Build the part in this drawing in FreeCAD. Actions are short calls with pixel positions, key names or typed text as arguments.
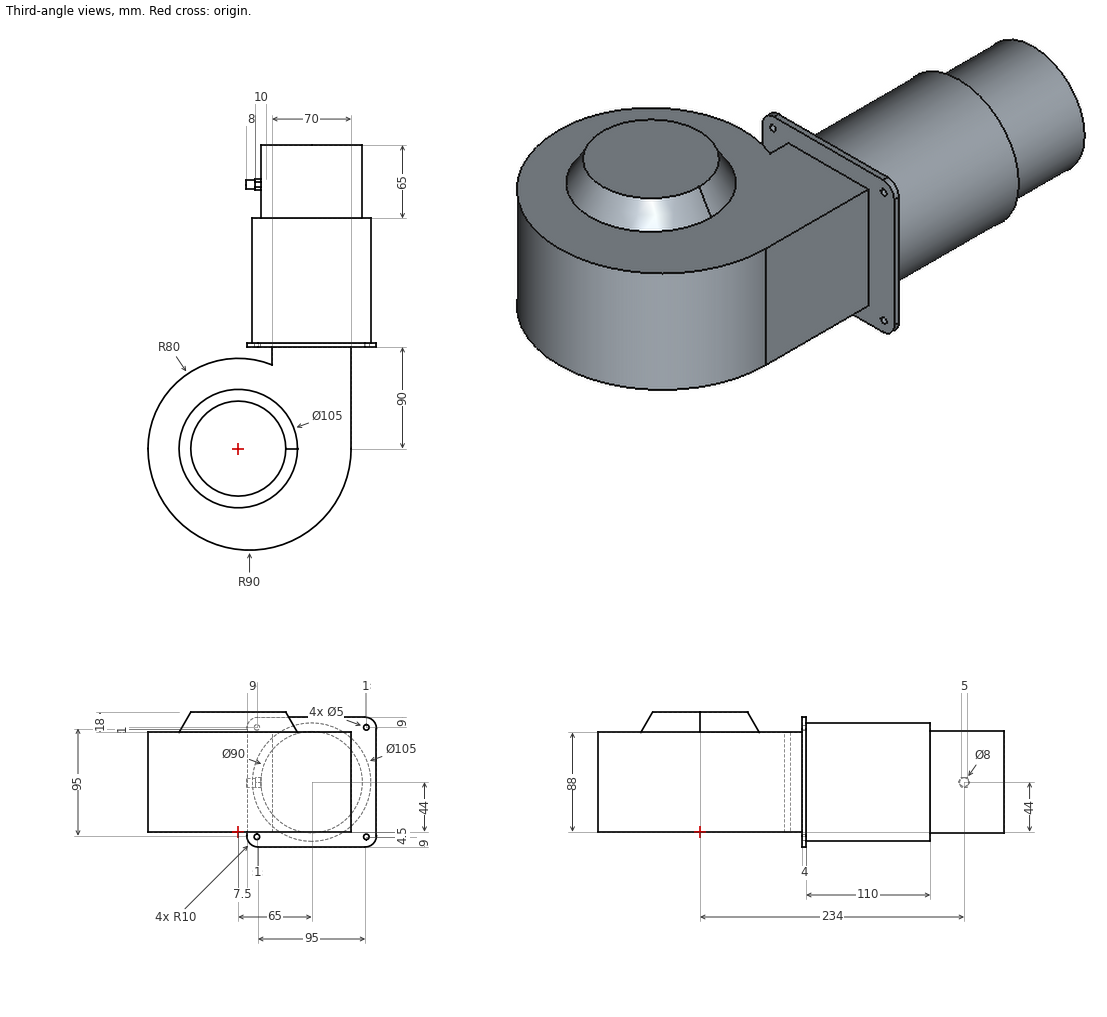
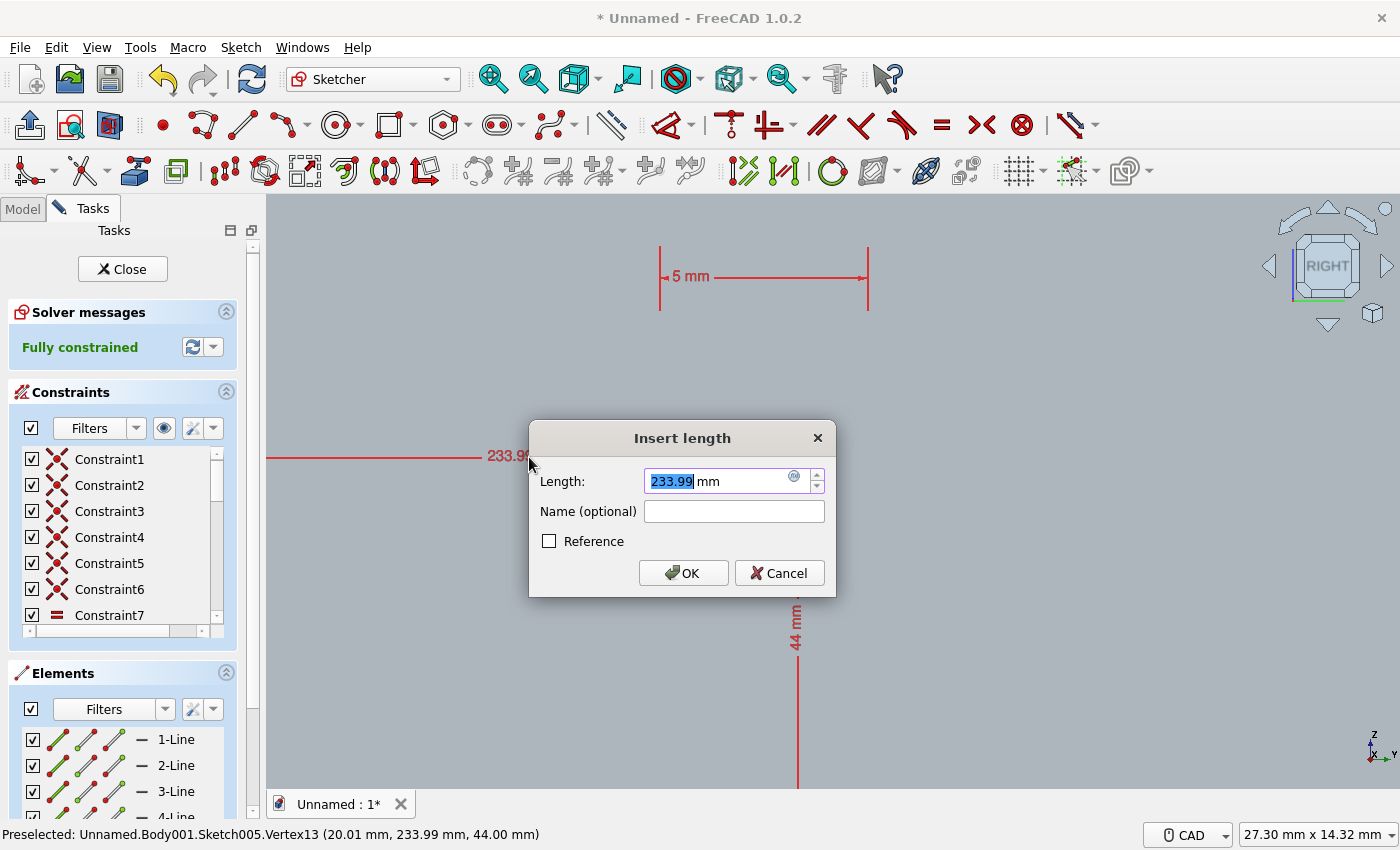
text(234)
key(Return)
key(Escape)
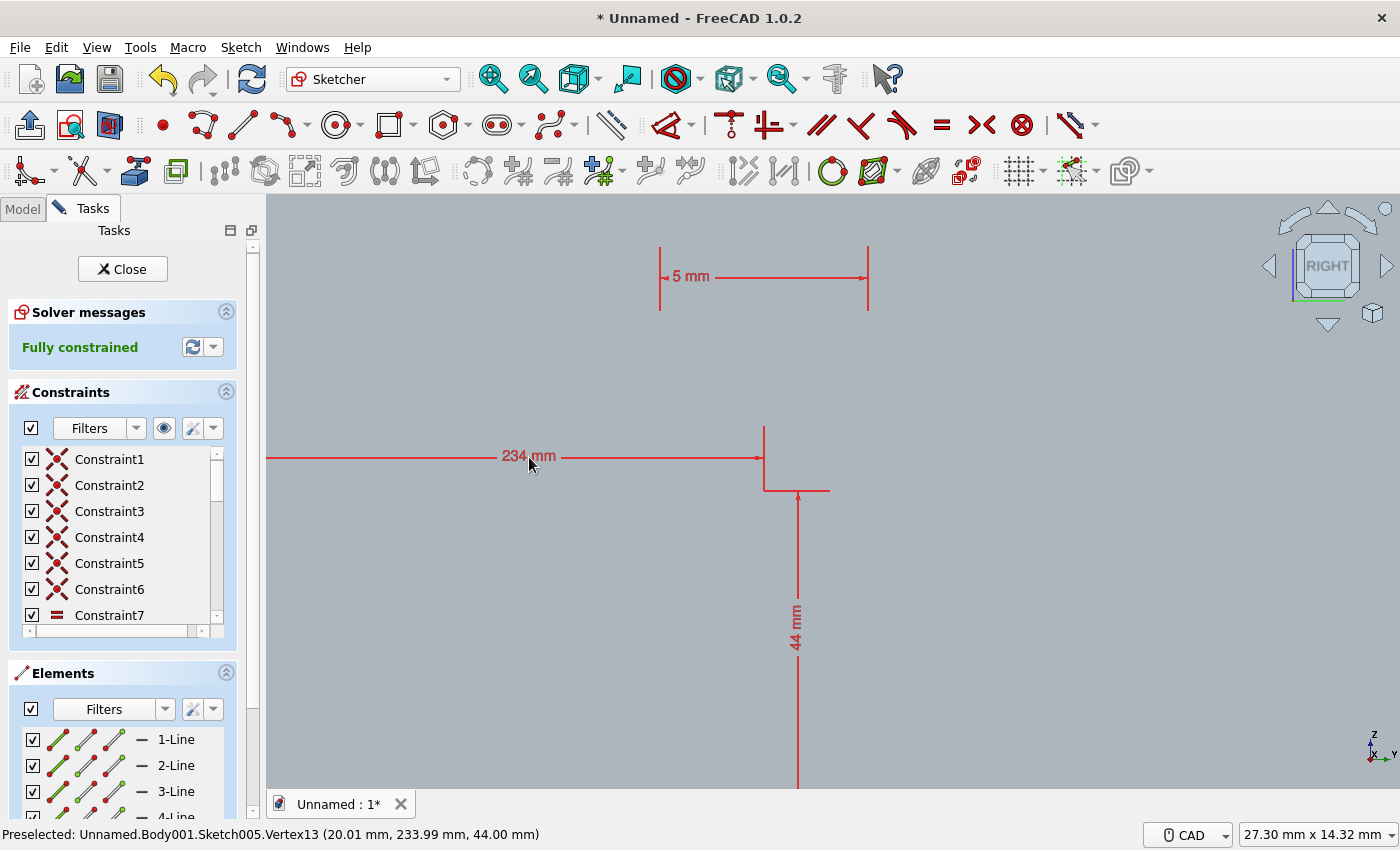
click(123, 269)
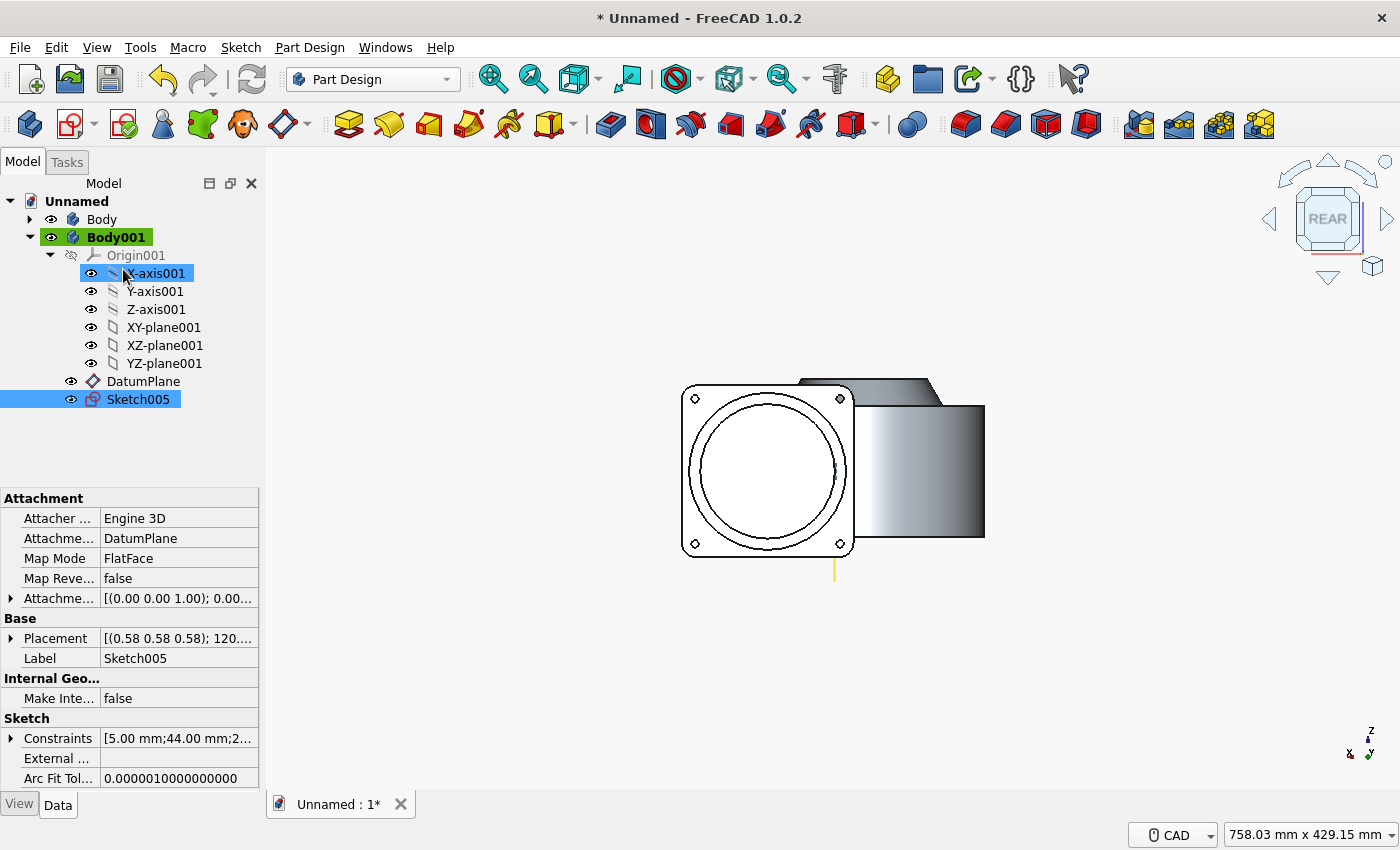
click(350, 124)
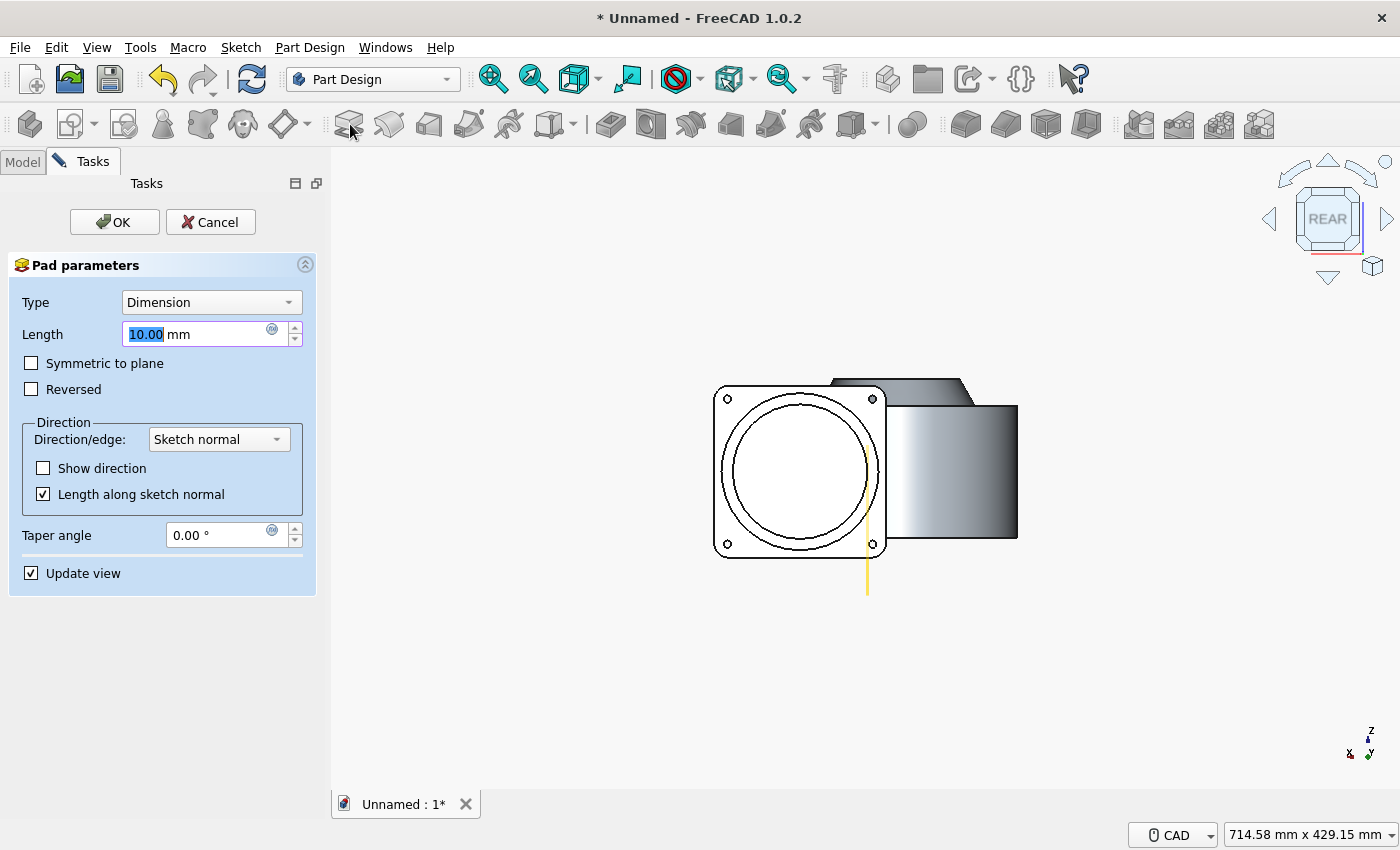
text(10)
key(Tab)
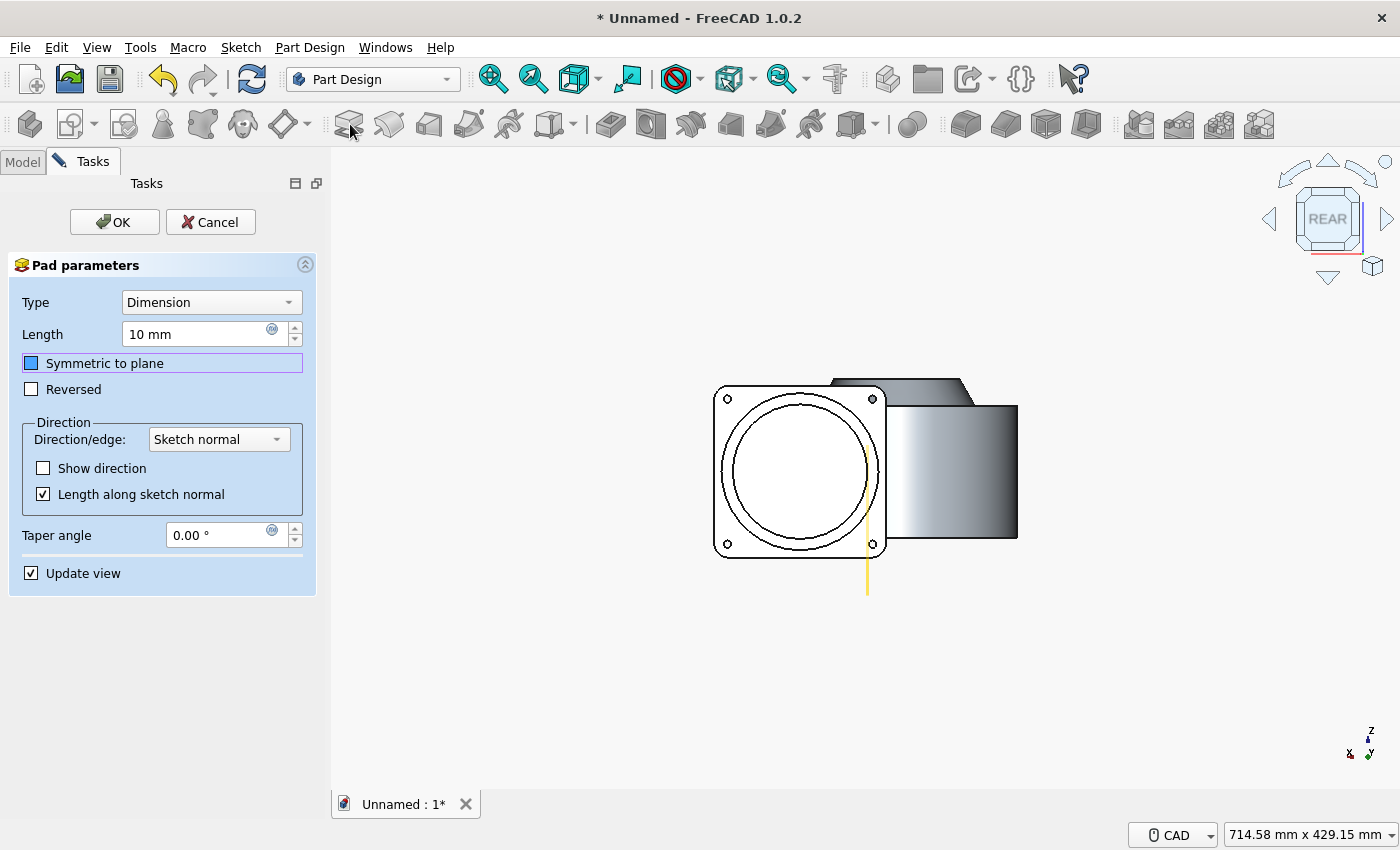
click(30, 363)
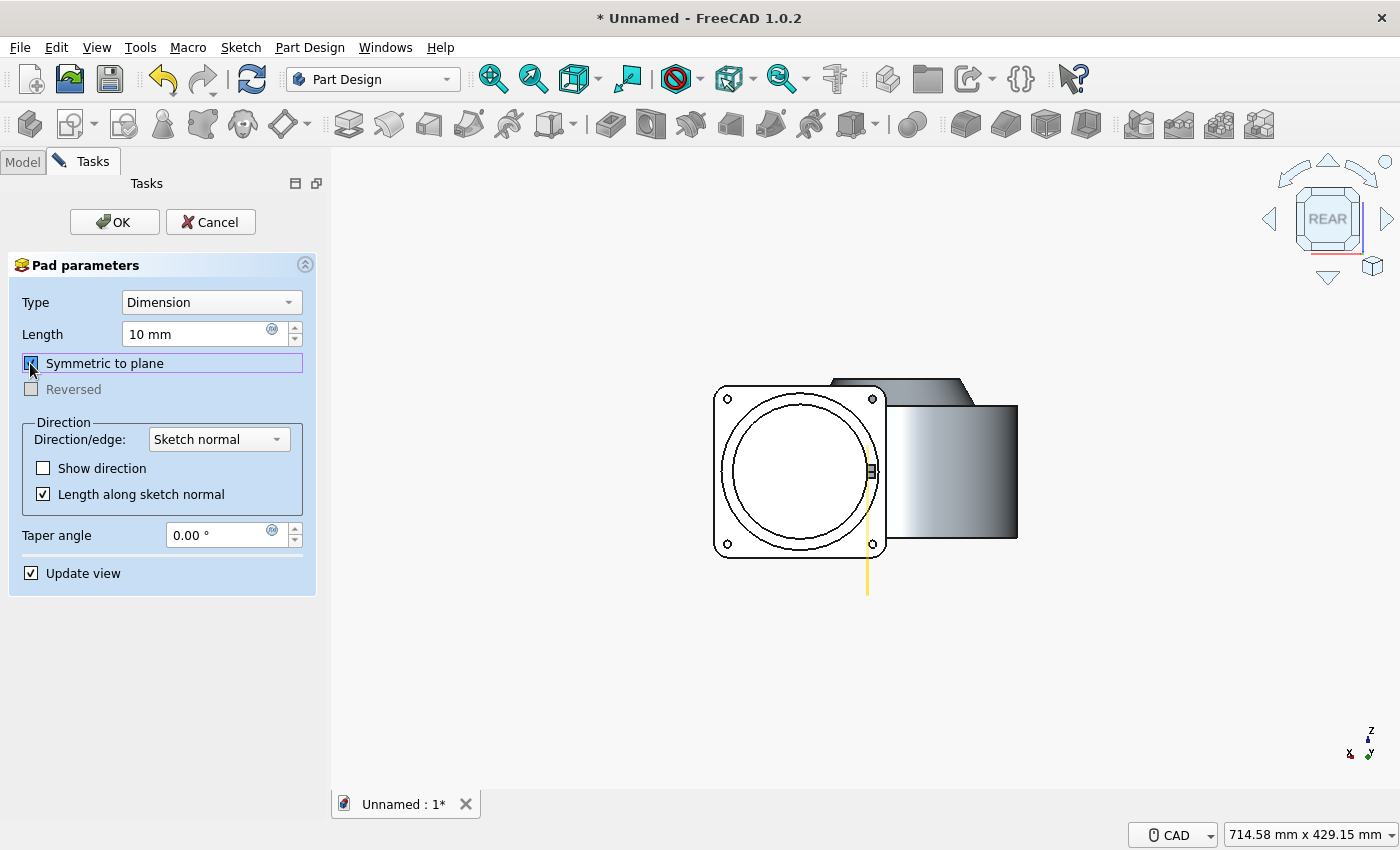
click(115, 222)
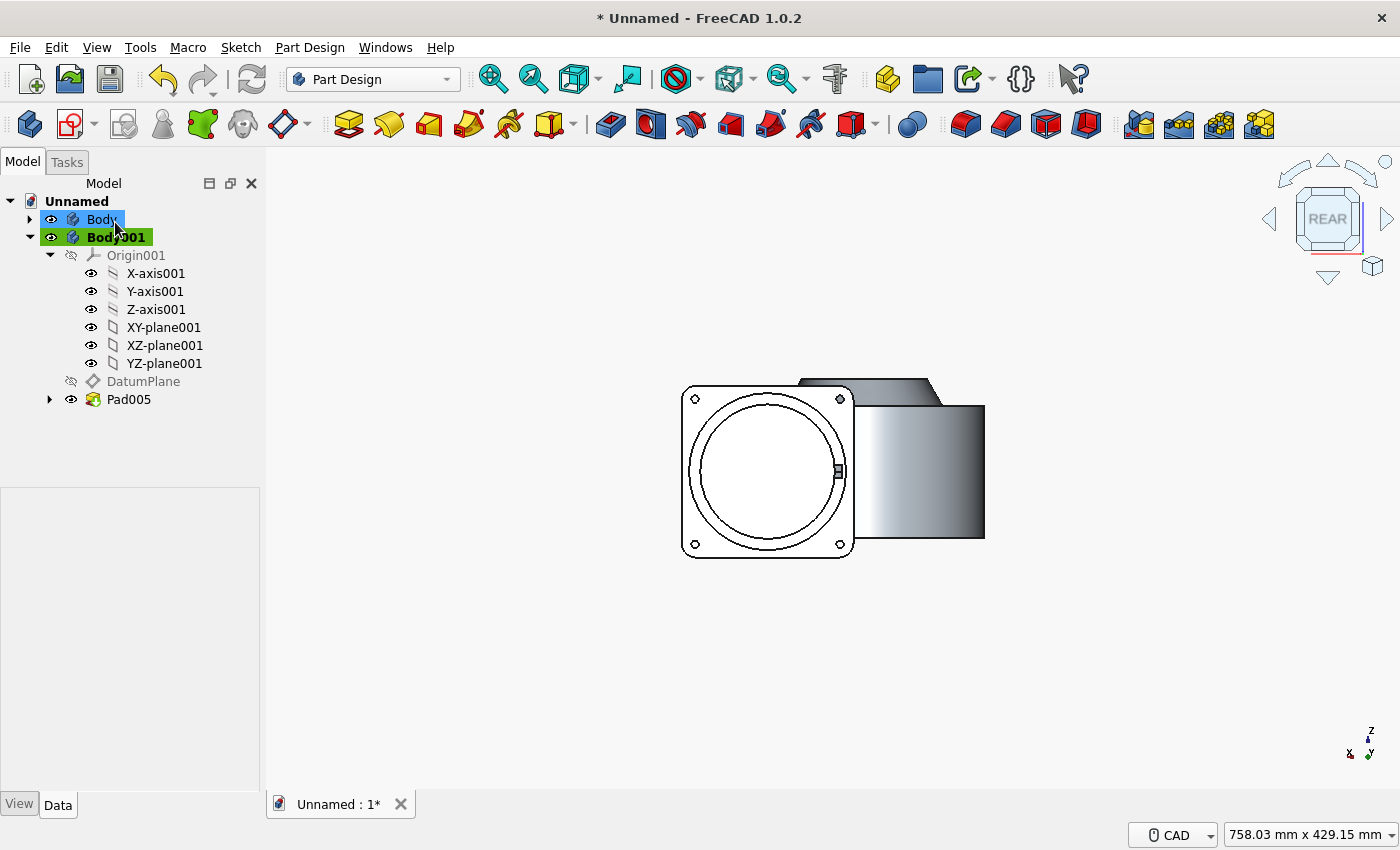
key(v)
key(f)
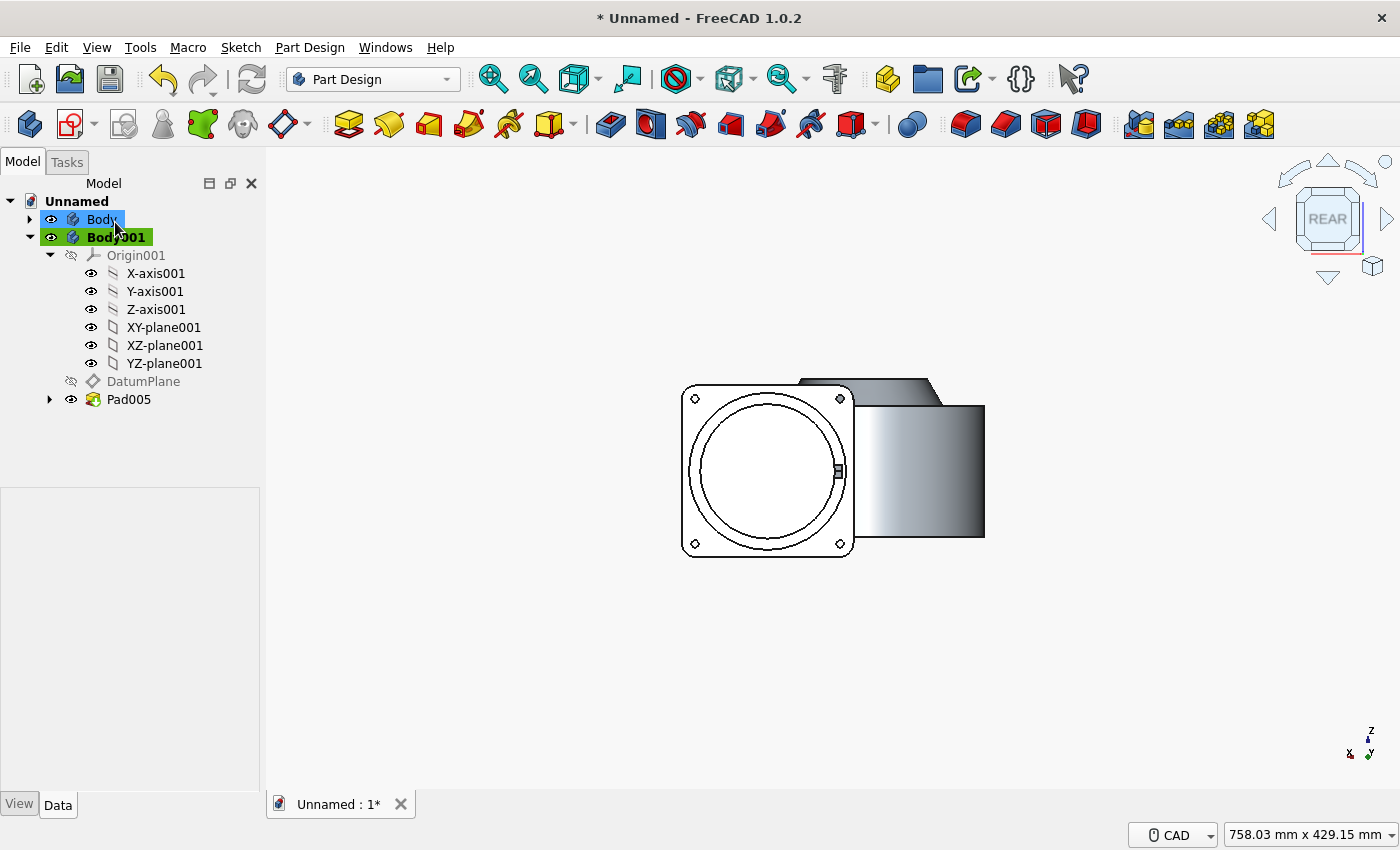
double_click(96, 219)